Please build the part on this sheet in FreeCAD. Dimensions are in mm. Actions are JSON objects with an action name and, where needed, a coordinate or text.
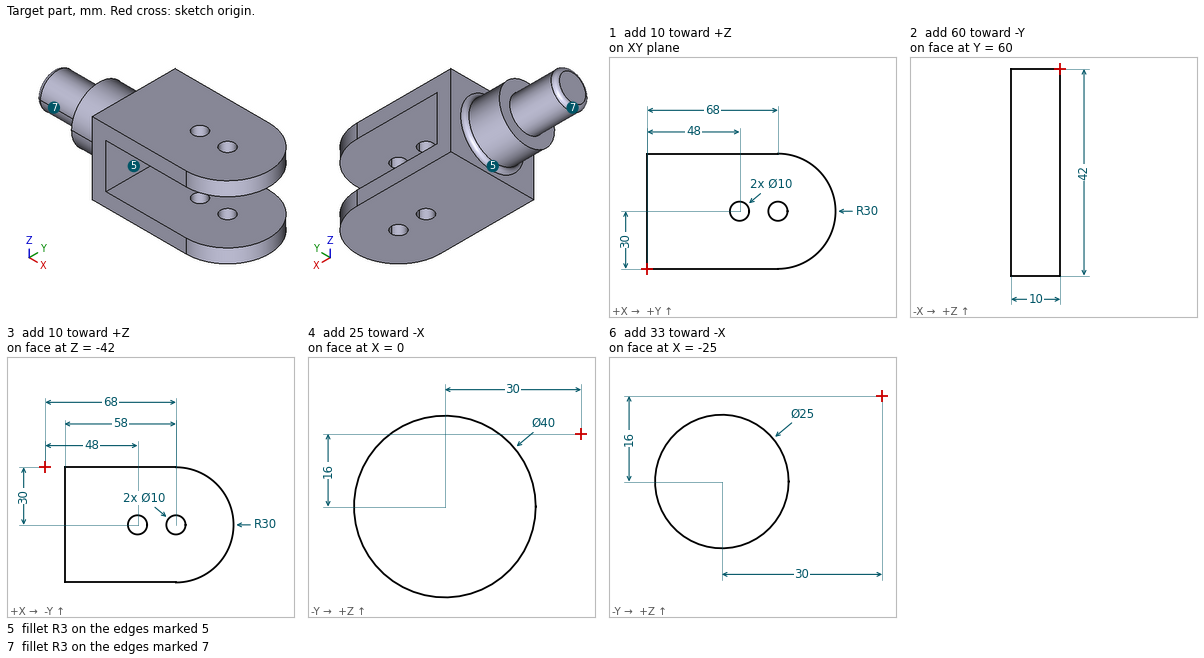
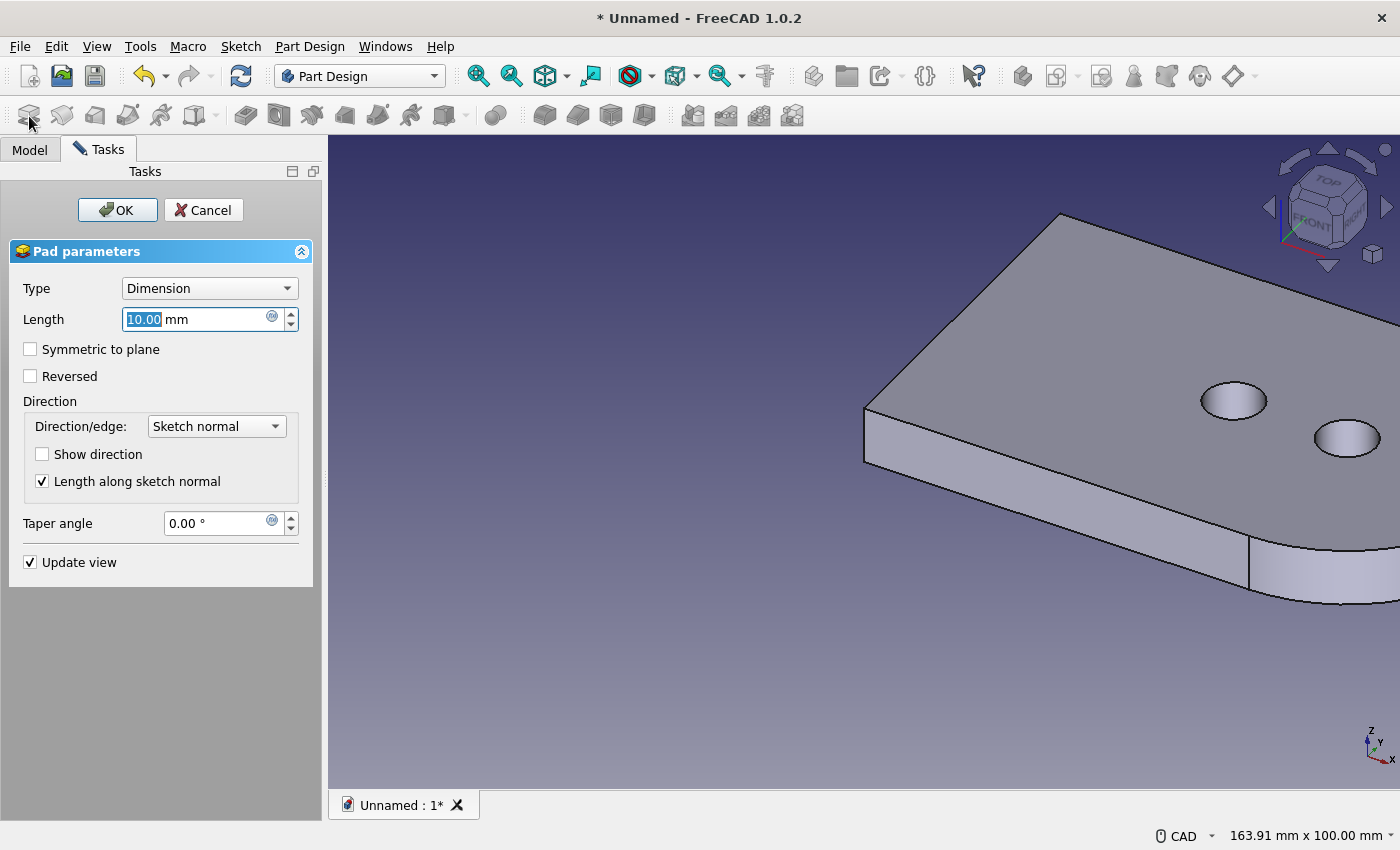
{"action": "type", "text": "10"}
{"action": "key", "text": "Tab"}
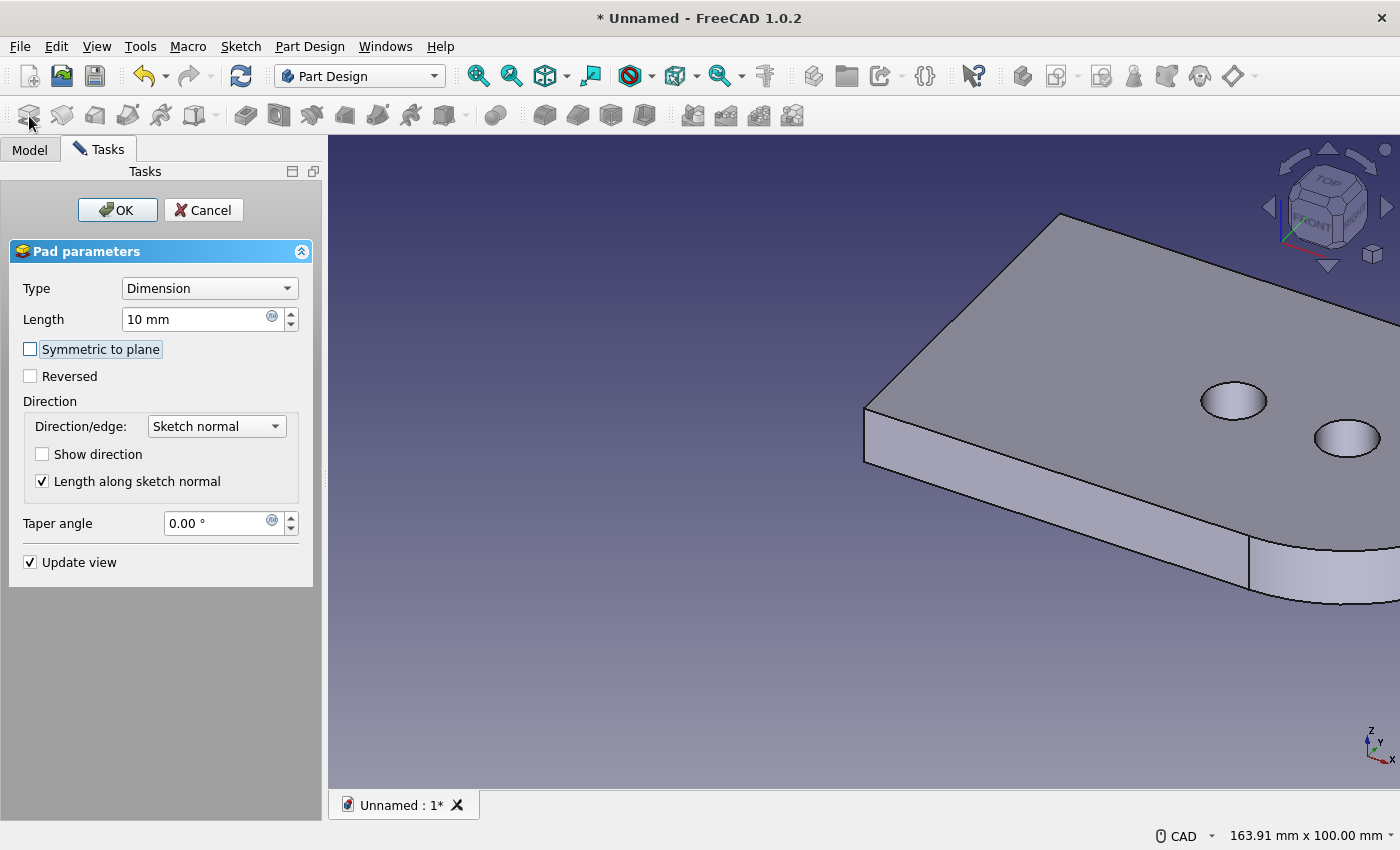
{"action": "left_click", "coordinate": [118, 210]}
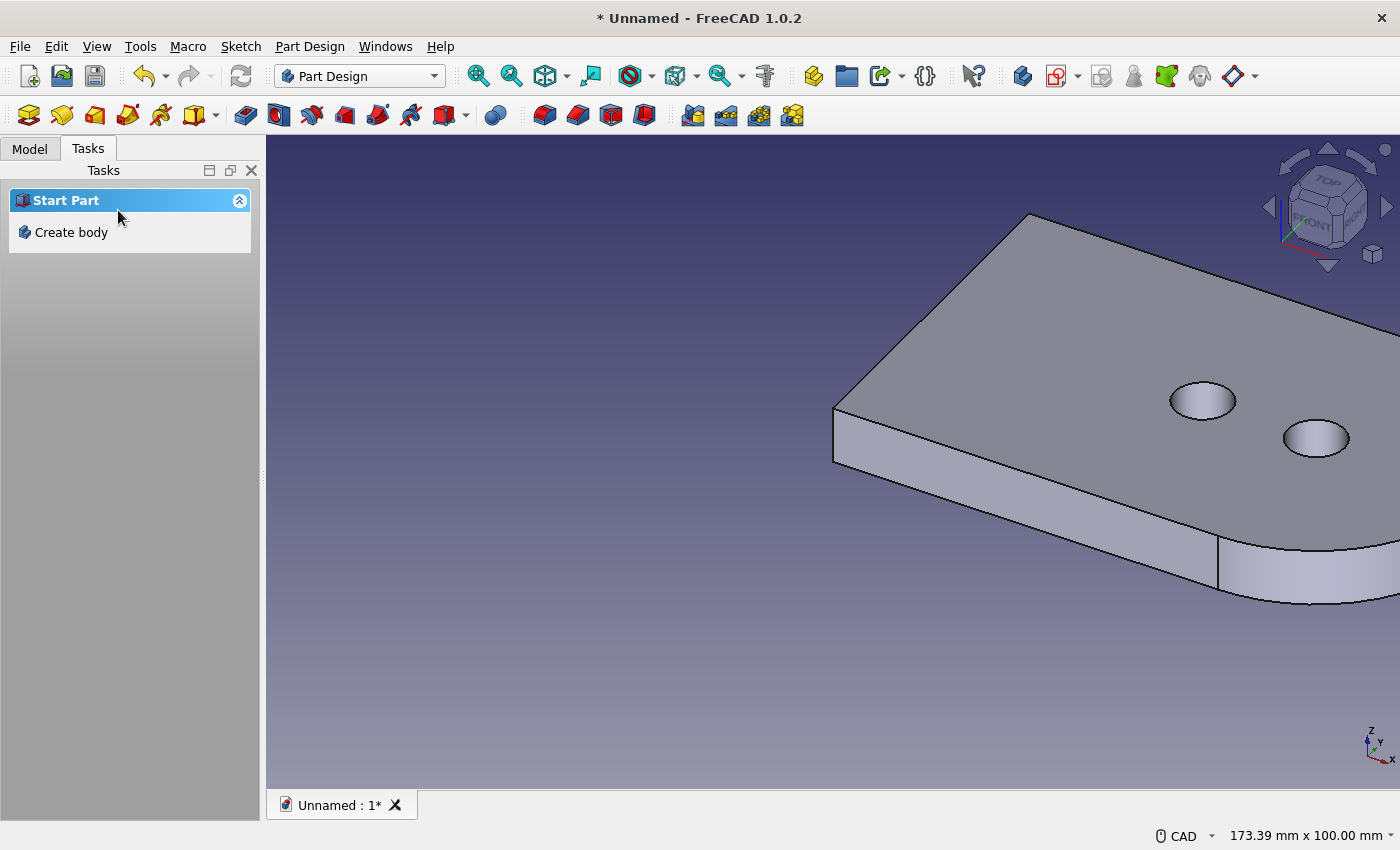
{"action": "key", "text": "v f"}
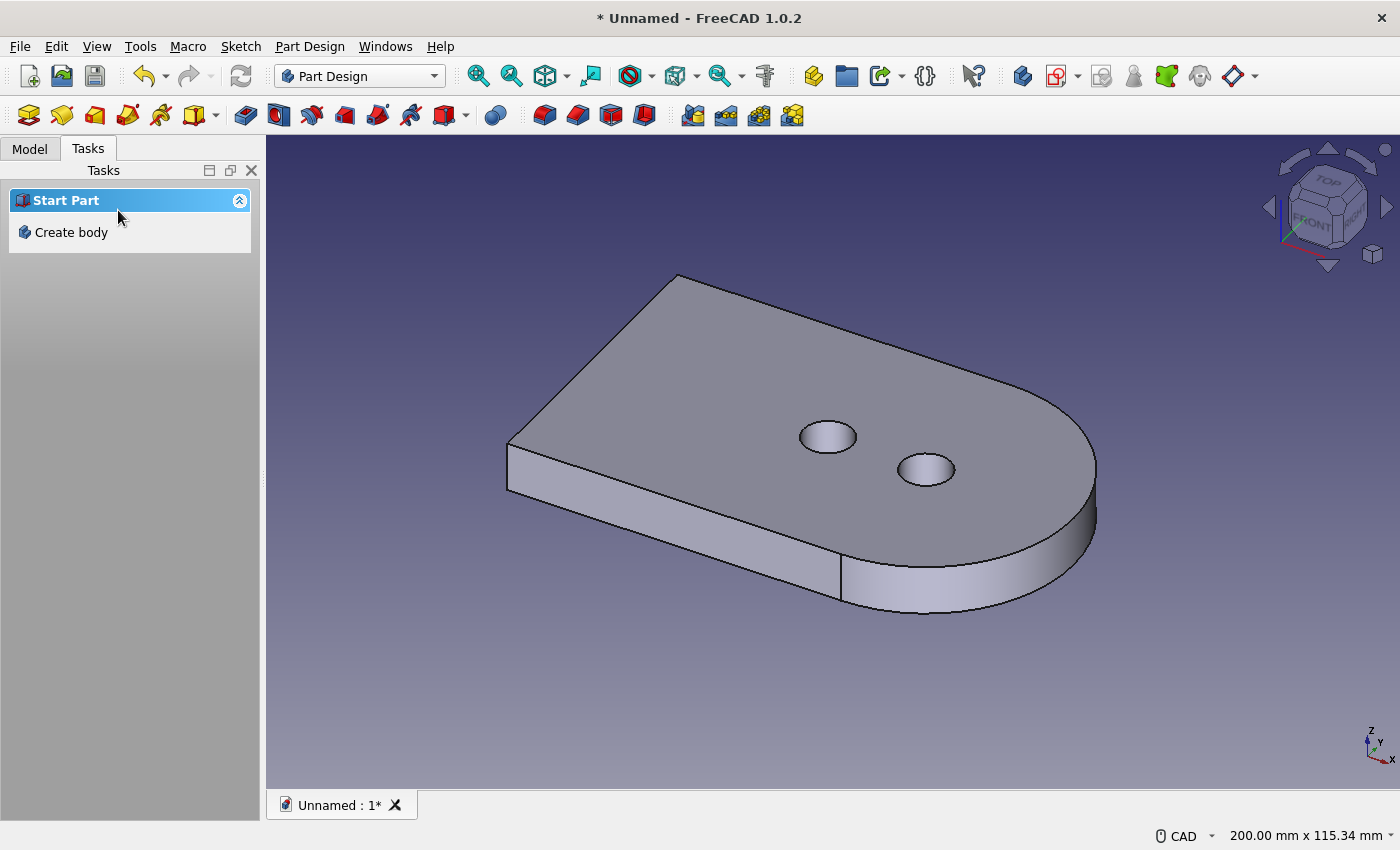
{"action": "key", "text": "4"}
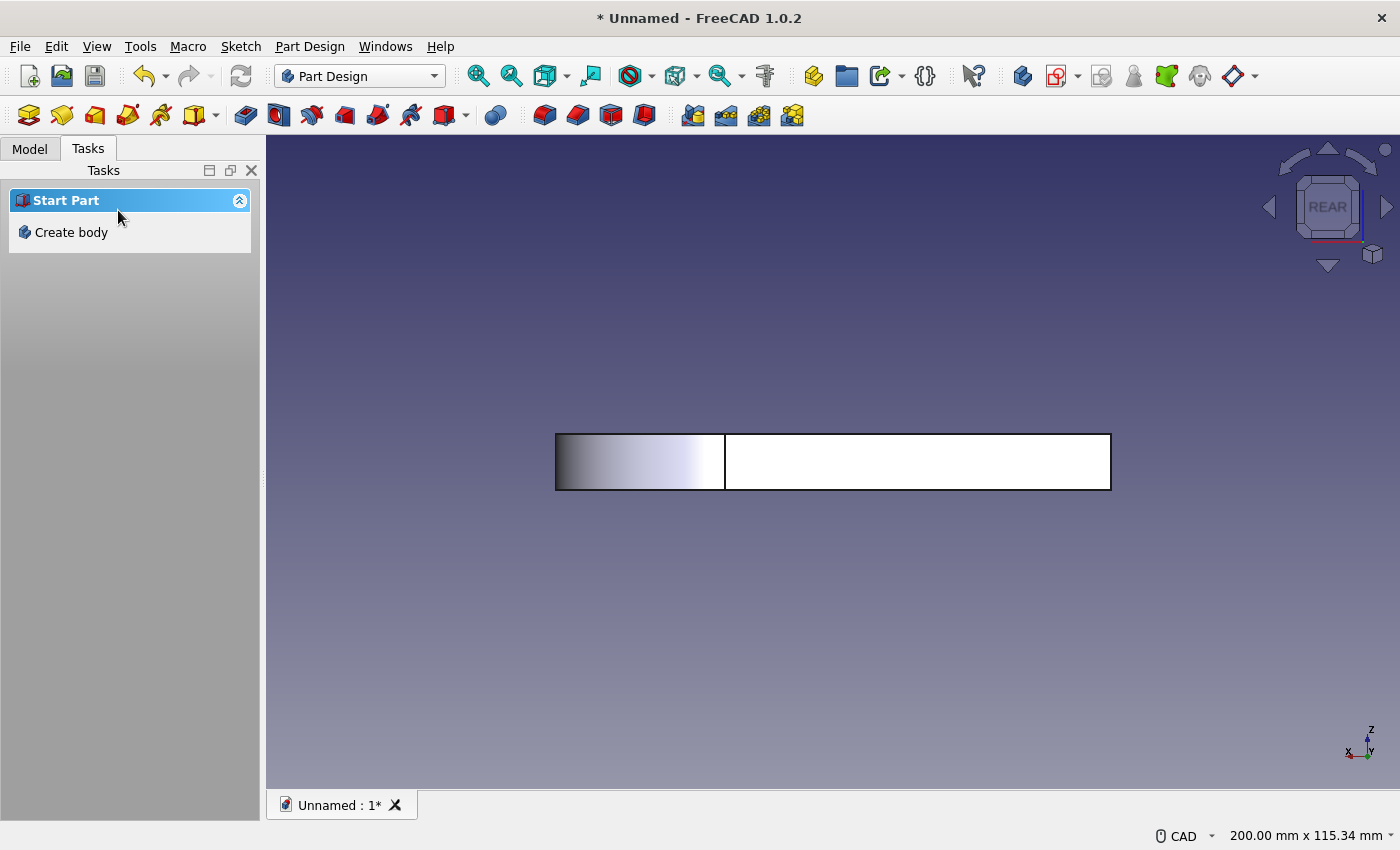
{"action": "left_click", "coordinate": [808, 461]}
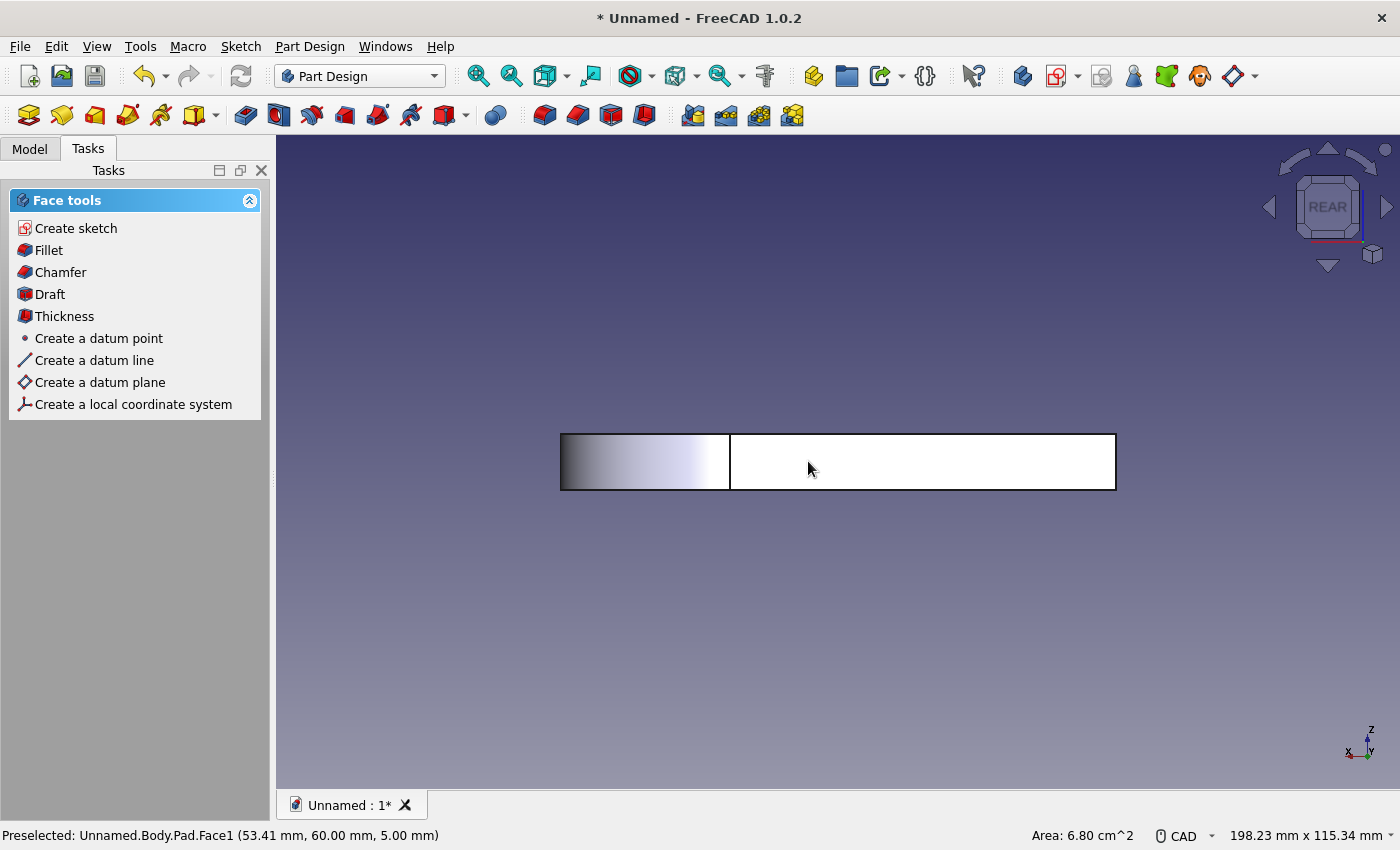
{"action": "left_click", "coordinate": [1056, 76]}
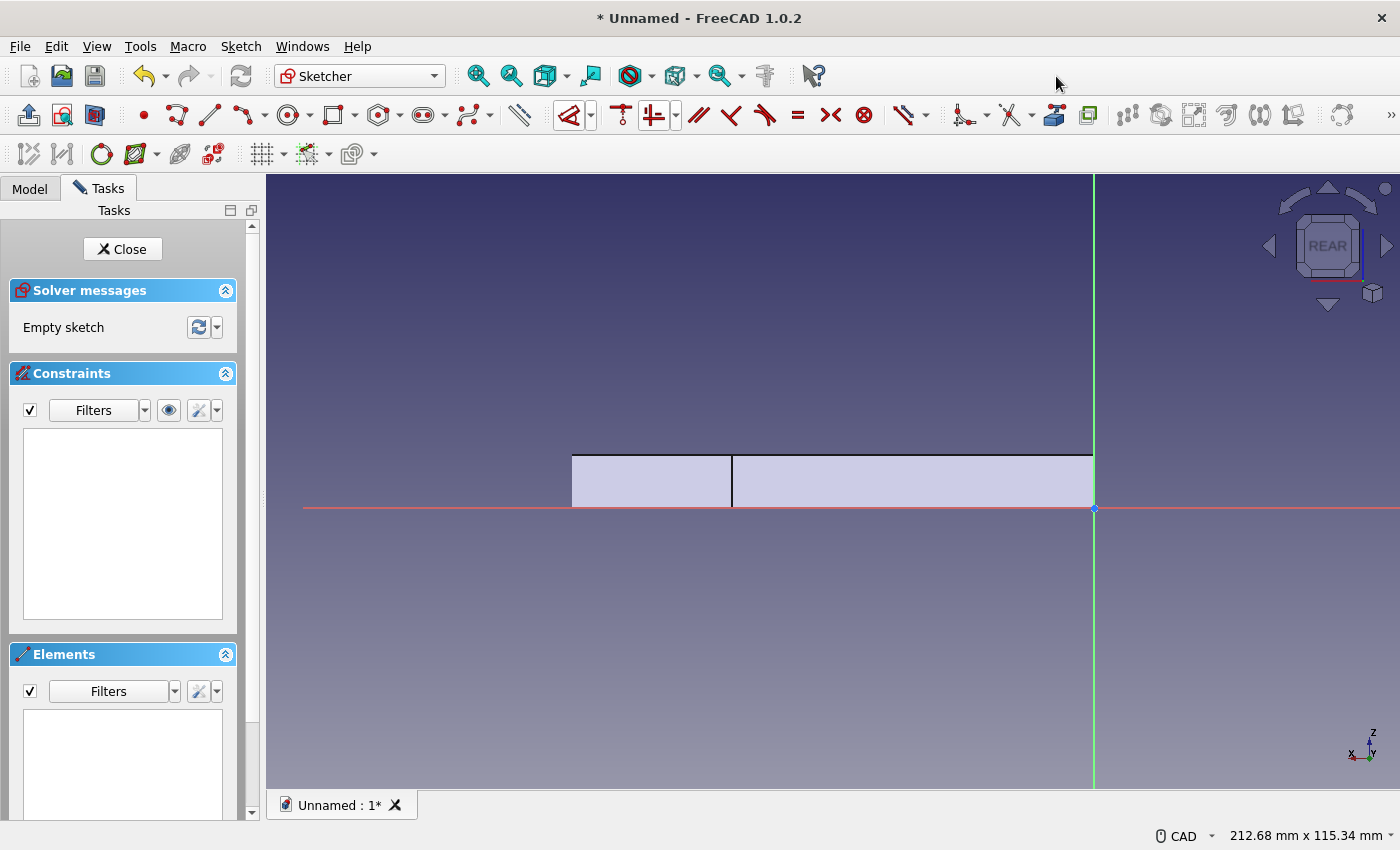
{"action": "scroll", "coordinate": [1235, 761], "scroll_direction": "up", "scroll_amount": 3}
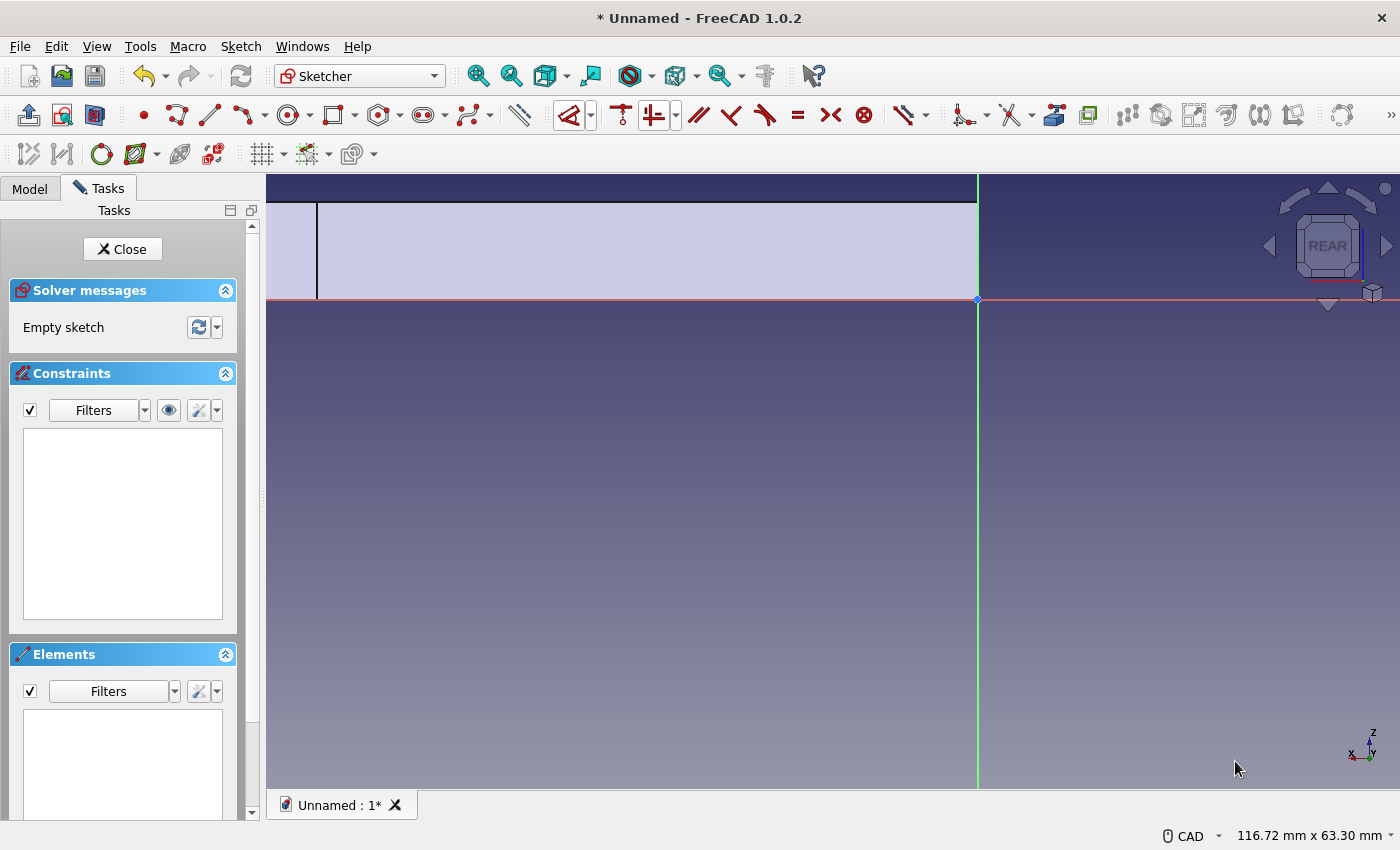
{"action": "key", "text": "g r"}